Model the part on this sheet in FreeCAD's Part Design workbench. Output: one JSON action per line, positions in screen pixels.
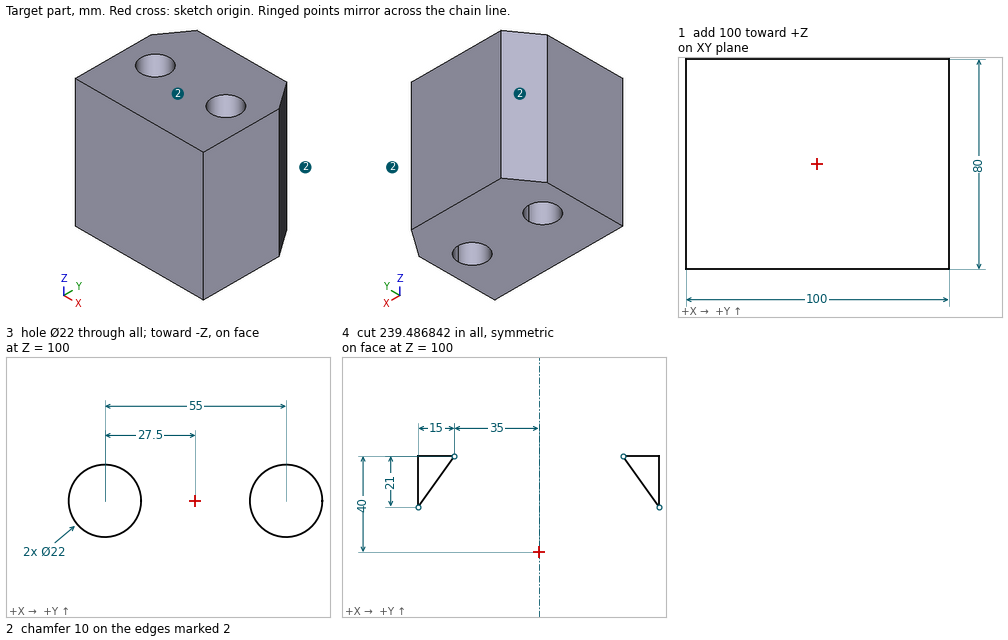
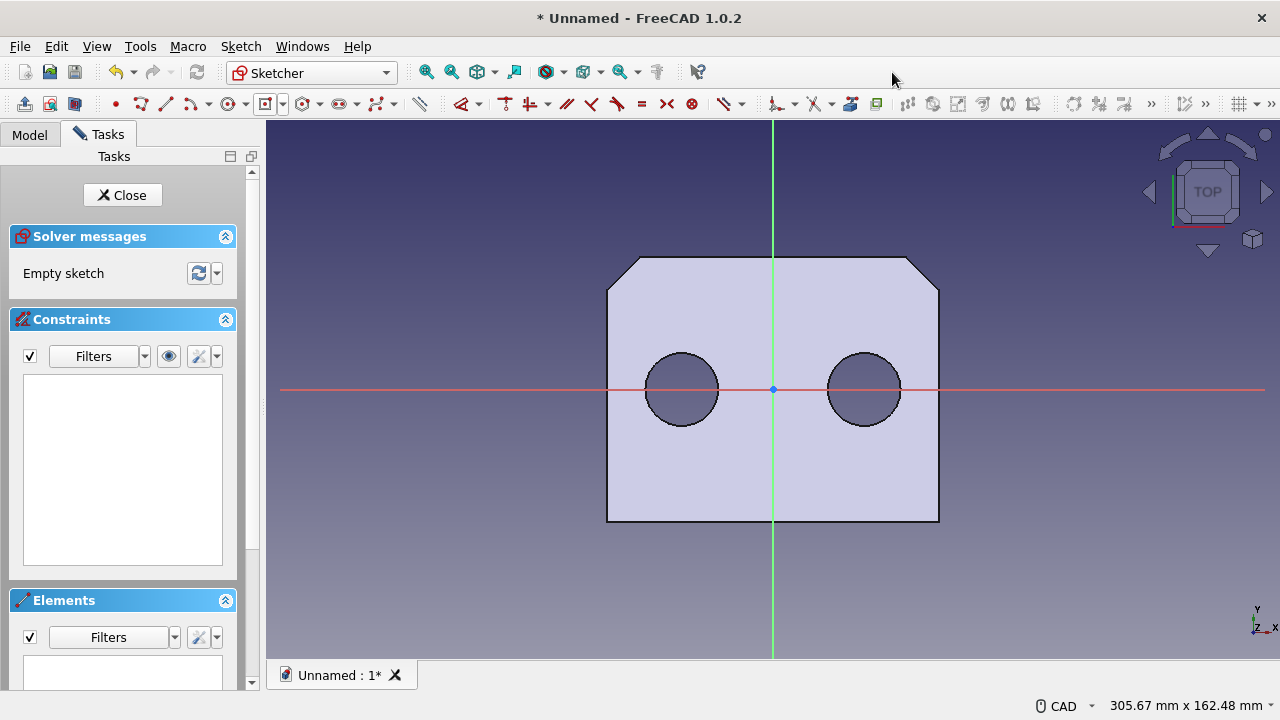
{"action": "scroll", "coordinate": [856, 242], "scroll_direction": "up", "scroll_amount": 3}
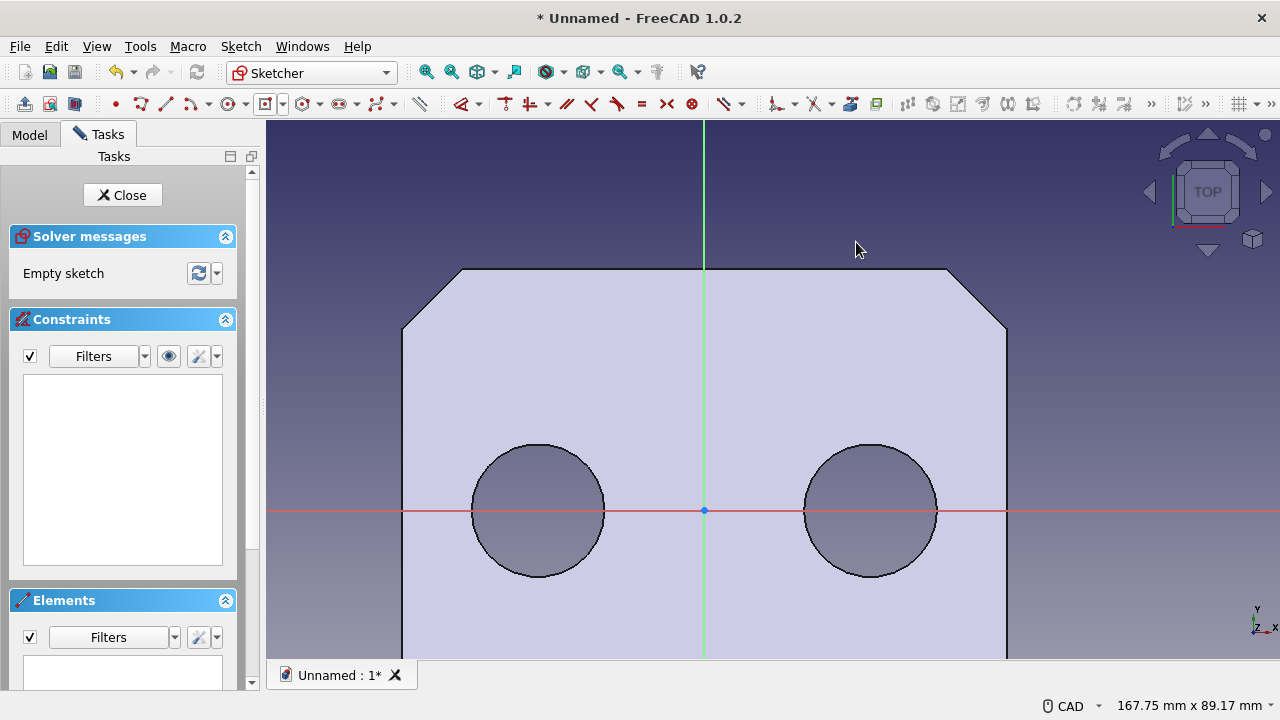
{"action": "left_click", "coordinate": [141, 104]}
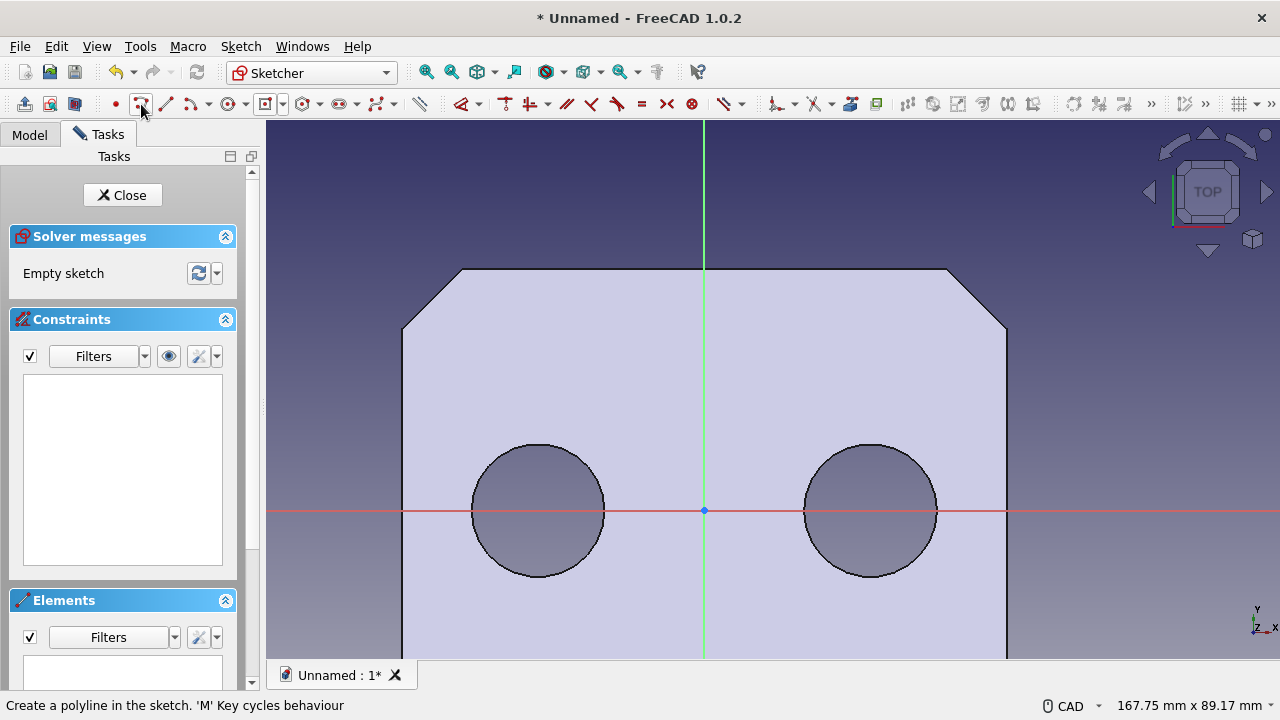
{"action": "left_click", "coordinate": [493, 269]}
{"action": "left_click", "coordinate": [402, 269]}
{"action": "left_click", "coordinate": [402, 396]}
{"action": "left_click", "coordinate": [493, 270]}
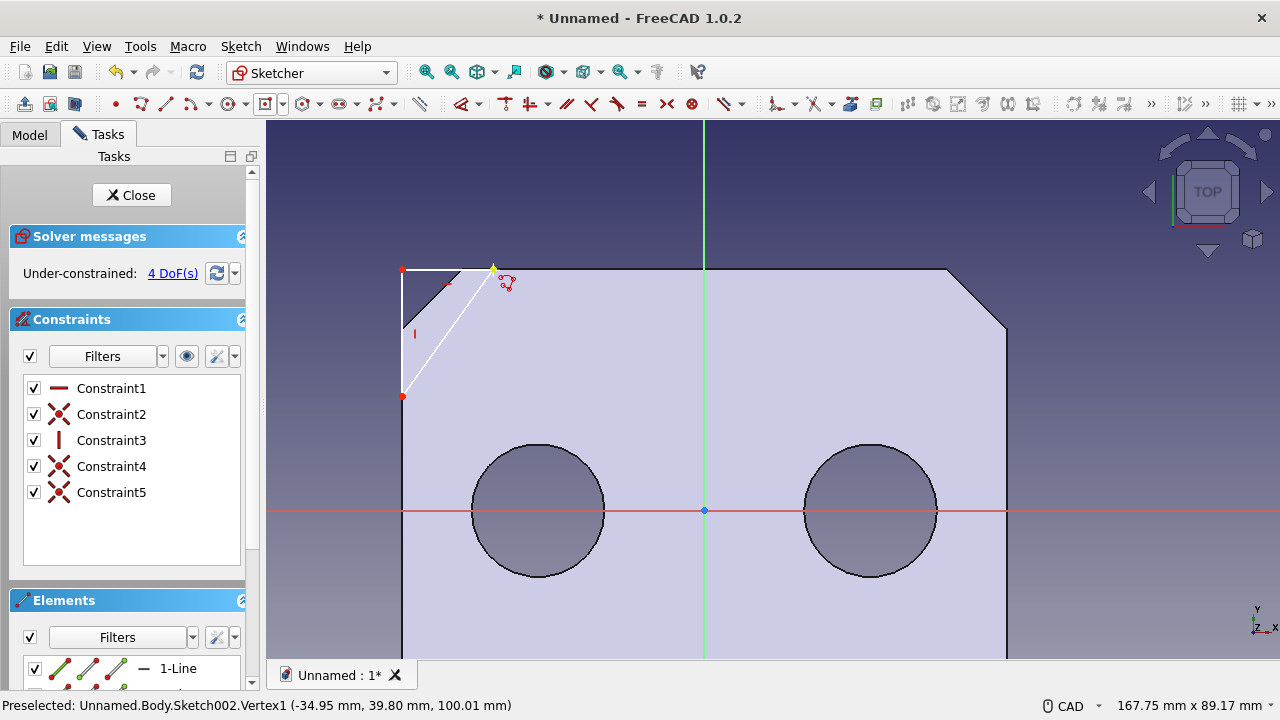
{"action": "left_click", "coordinate": [916, 269]}
{"action": "left_click", "coordinate": [1007, 396]}
{"action": "left_click", "coordinate": [1007, 269]}
{"action": "left_click", "coordinate": [916, 270]}
{"action": "key", "text": "Escape"}
{"action": "key", "text": "Escape"}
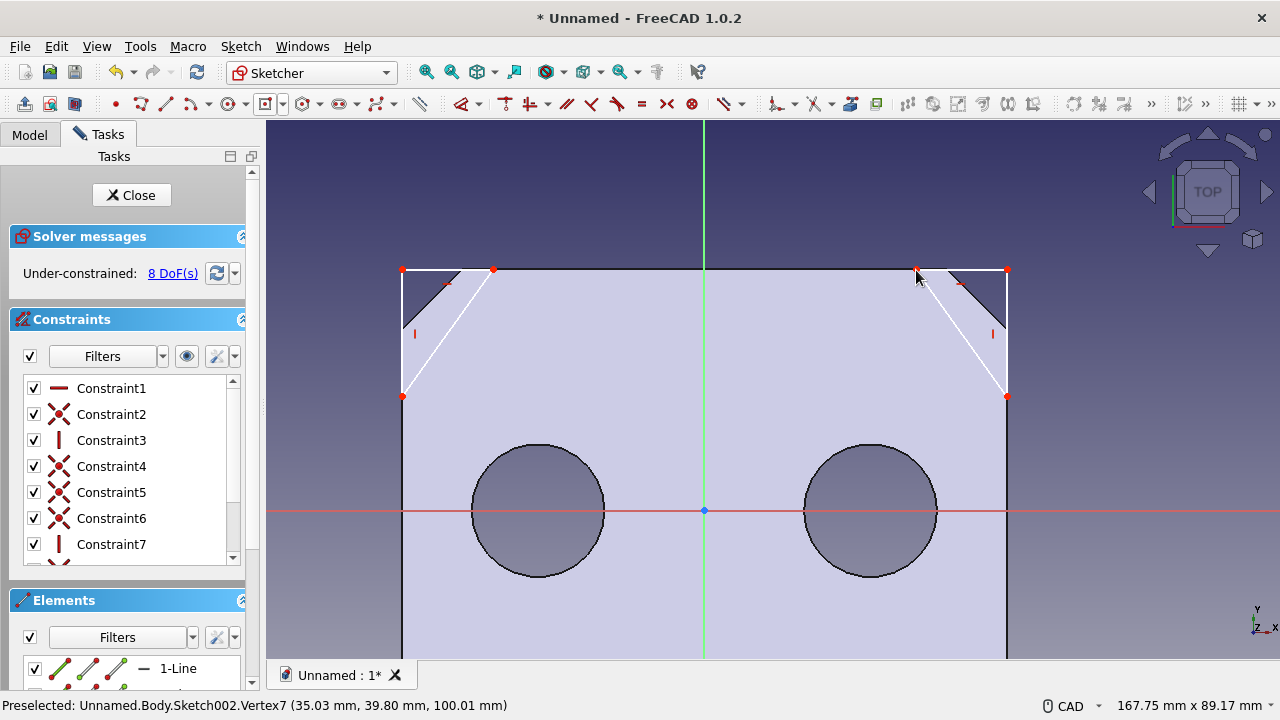
{"action": "left_click", "coordinate": [493, 270]}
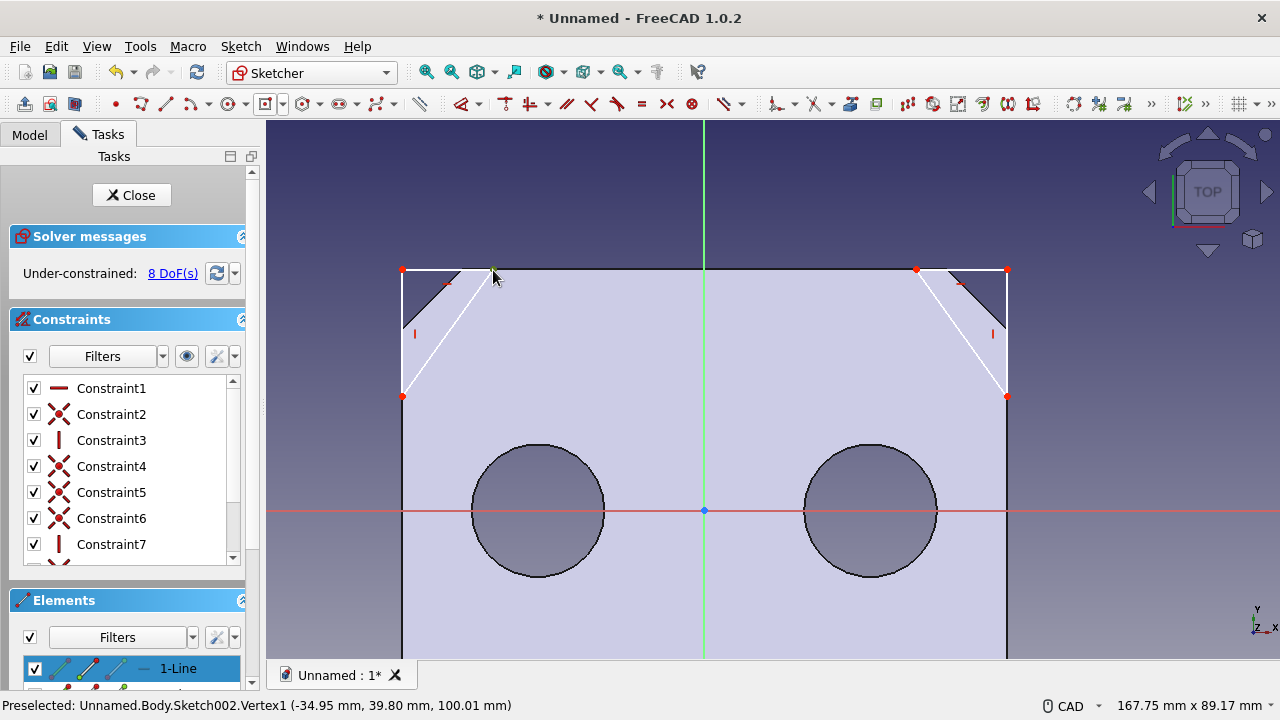
{"action": "left_click", "coordinate": [916, 270]}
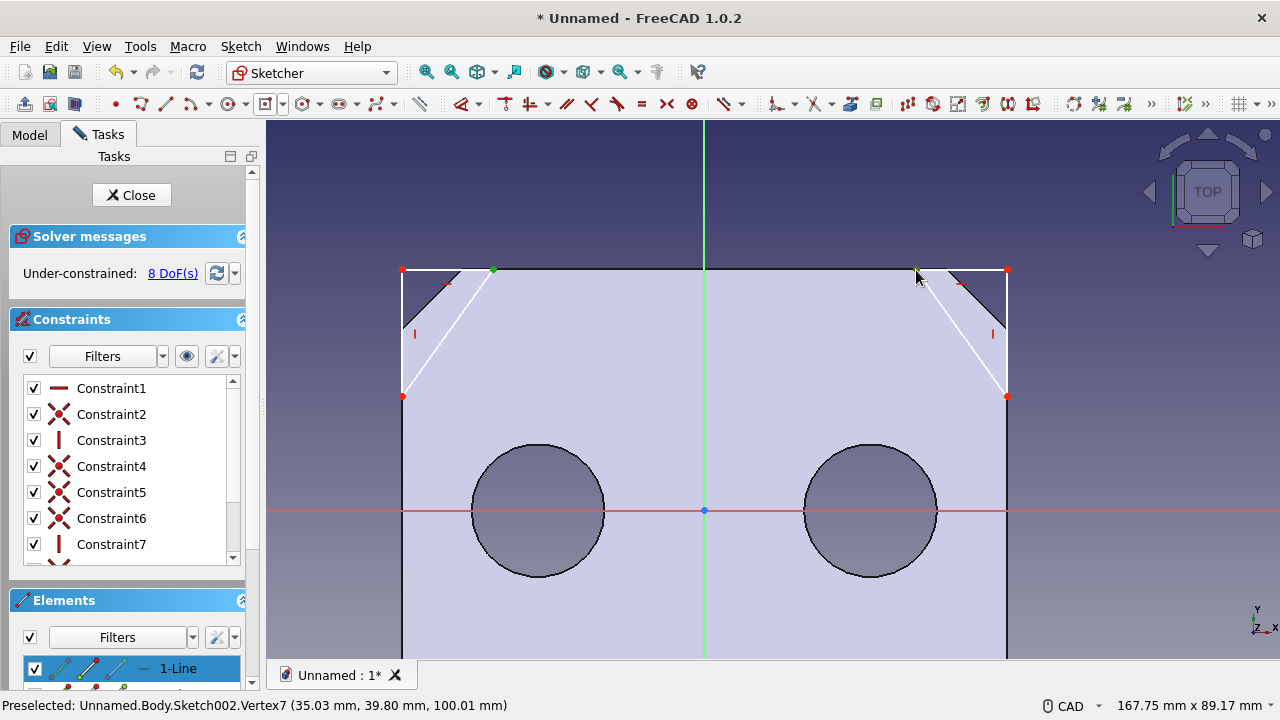
{"action": "left_click", "coordinate": [704, 596]}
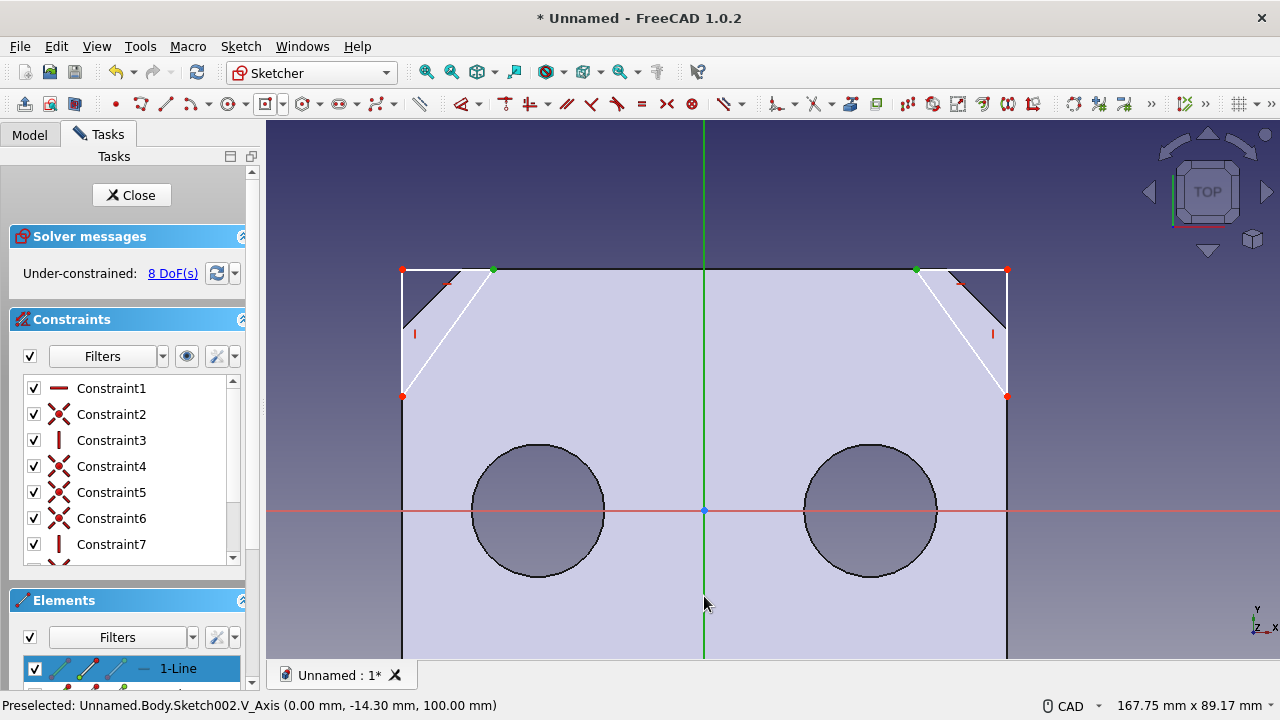
{"action": "left_click", "coordinate": [667, 104]}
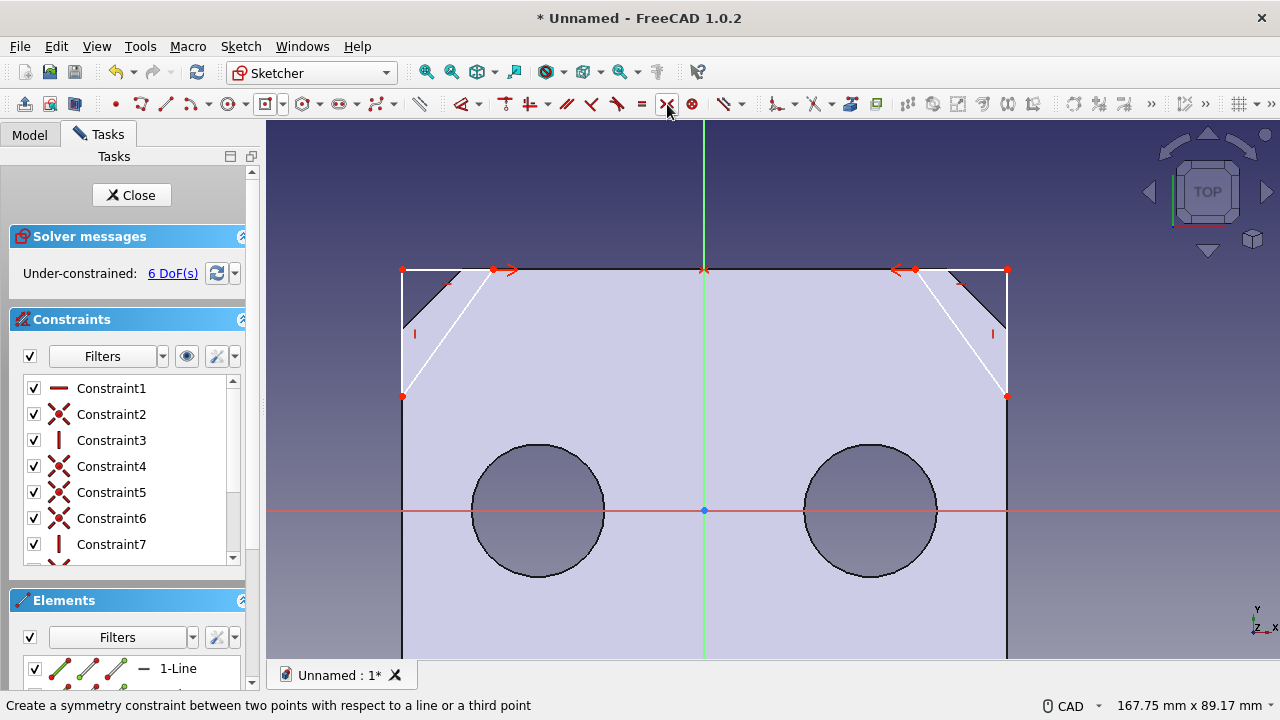
{"action": "left_click", "coordinate": [402, 397]}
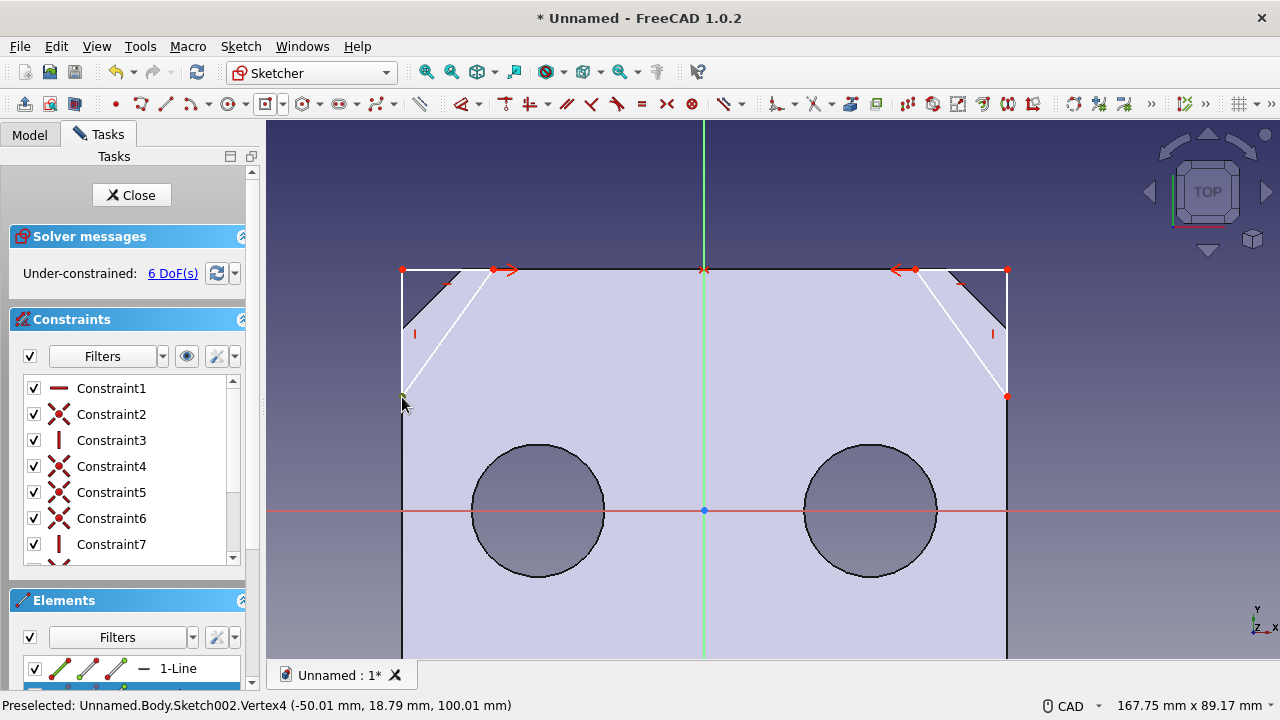
{"action": "left_click", "coordinate": [1007, 397]}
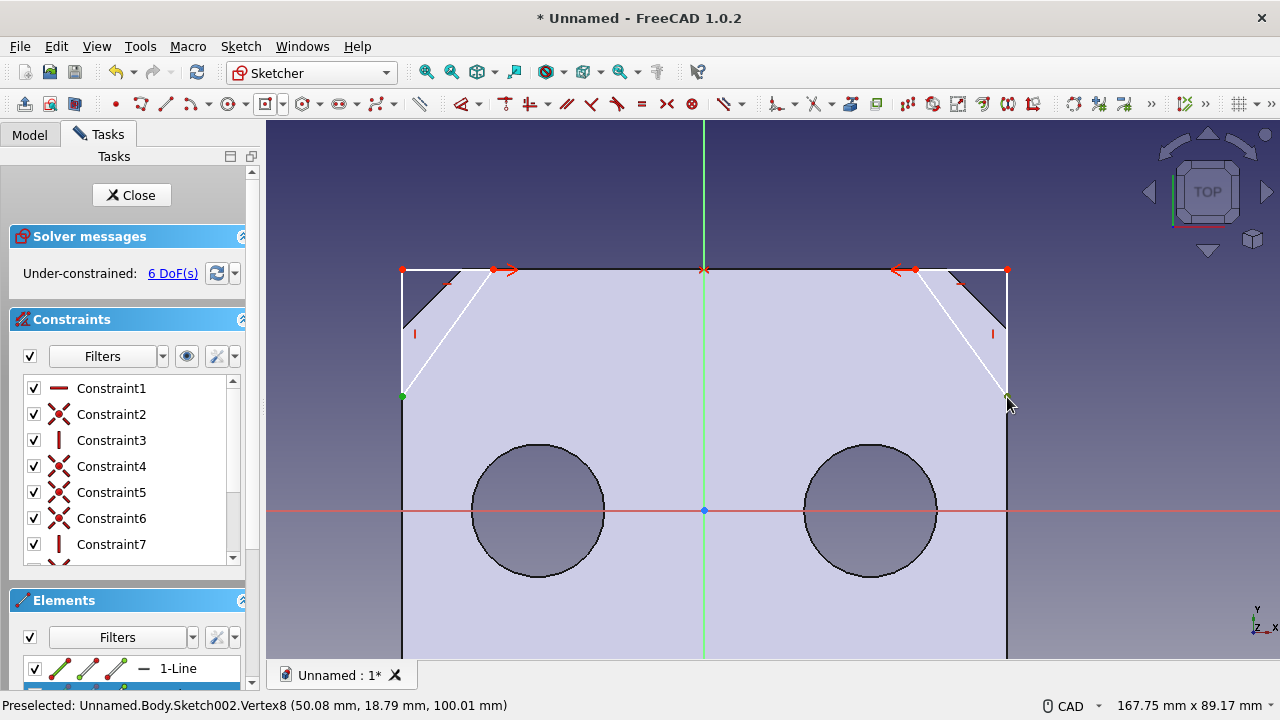
{"action": "left_click", "coordinate": [704, 596]}